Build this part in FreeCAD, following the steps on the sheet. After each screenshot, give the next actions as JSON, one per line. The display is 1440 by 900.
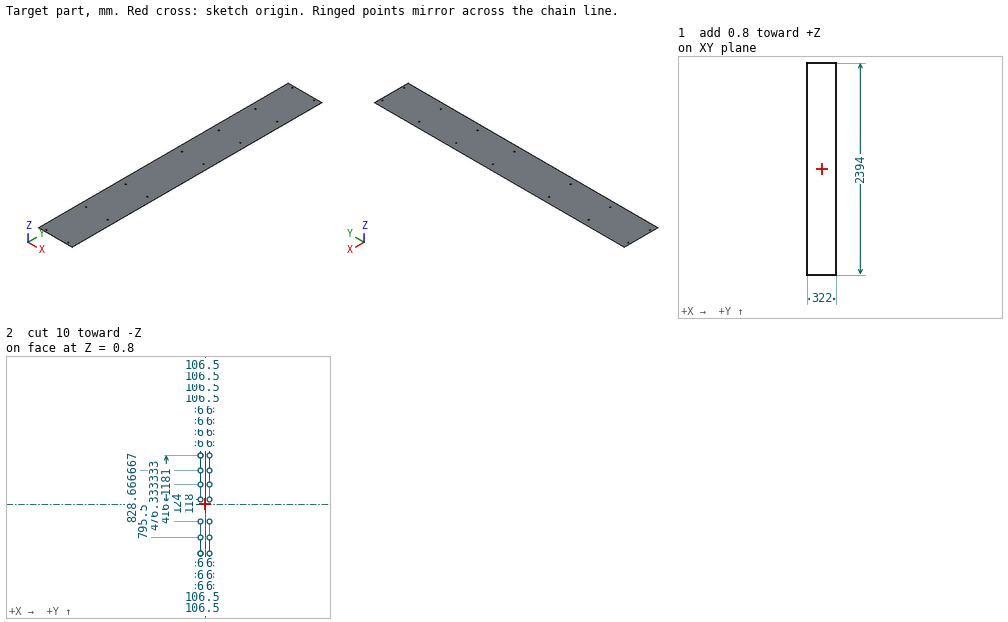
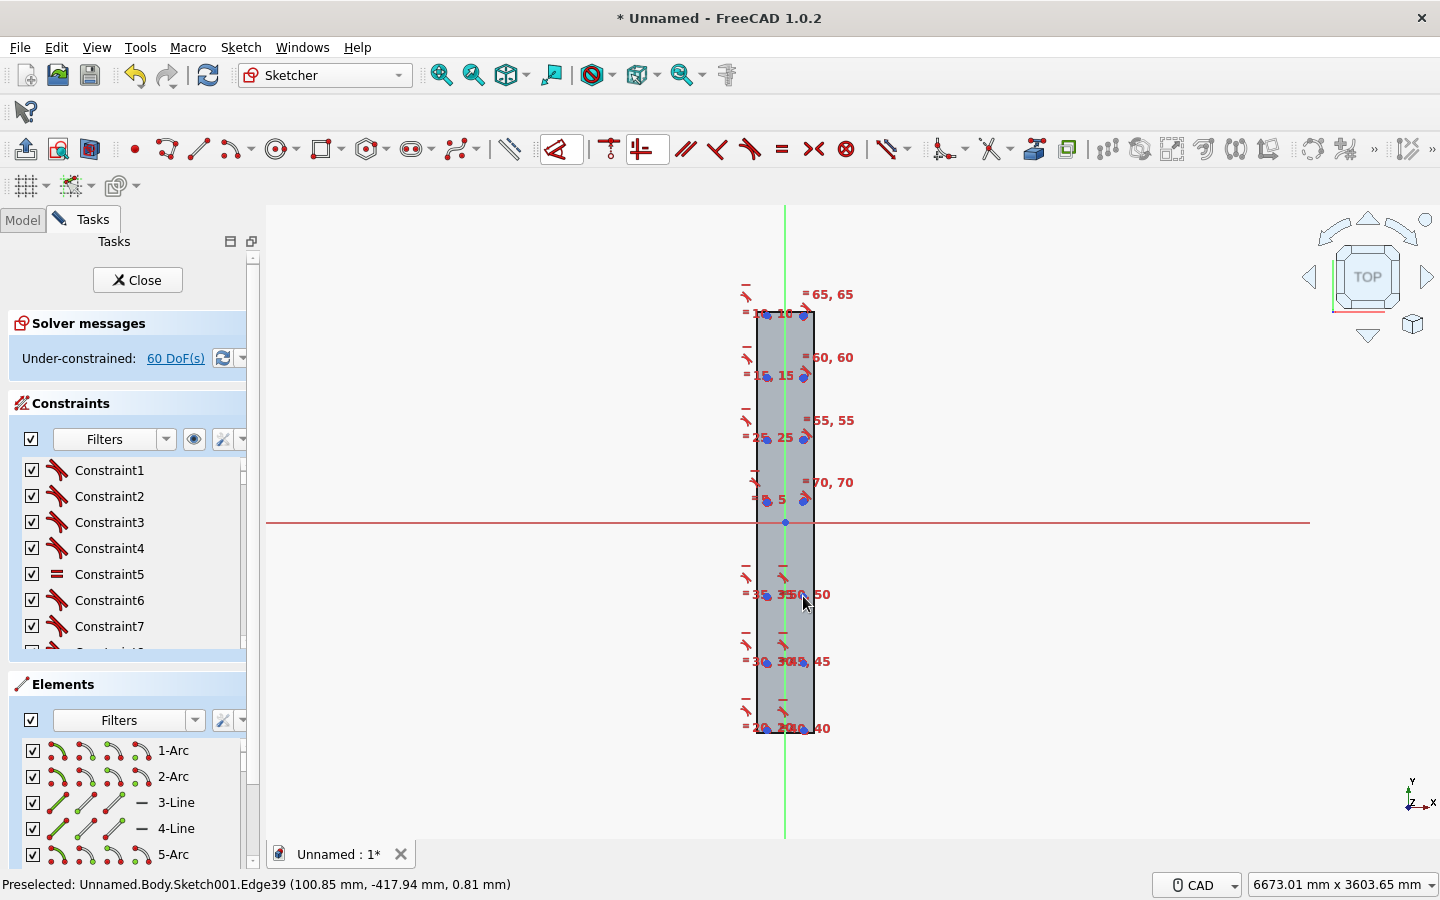
{"action": "scroll", "coordinate": [803, 439], "scroll_direction": "up", "scroll_amount": 14}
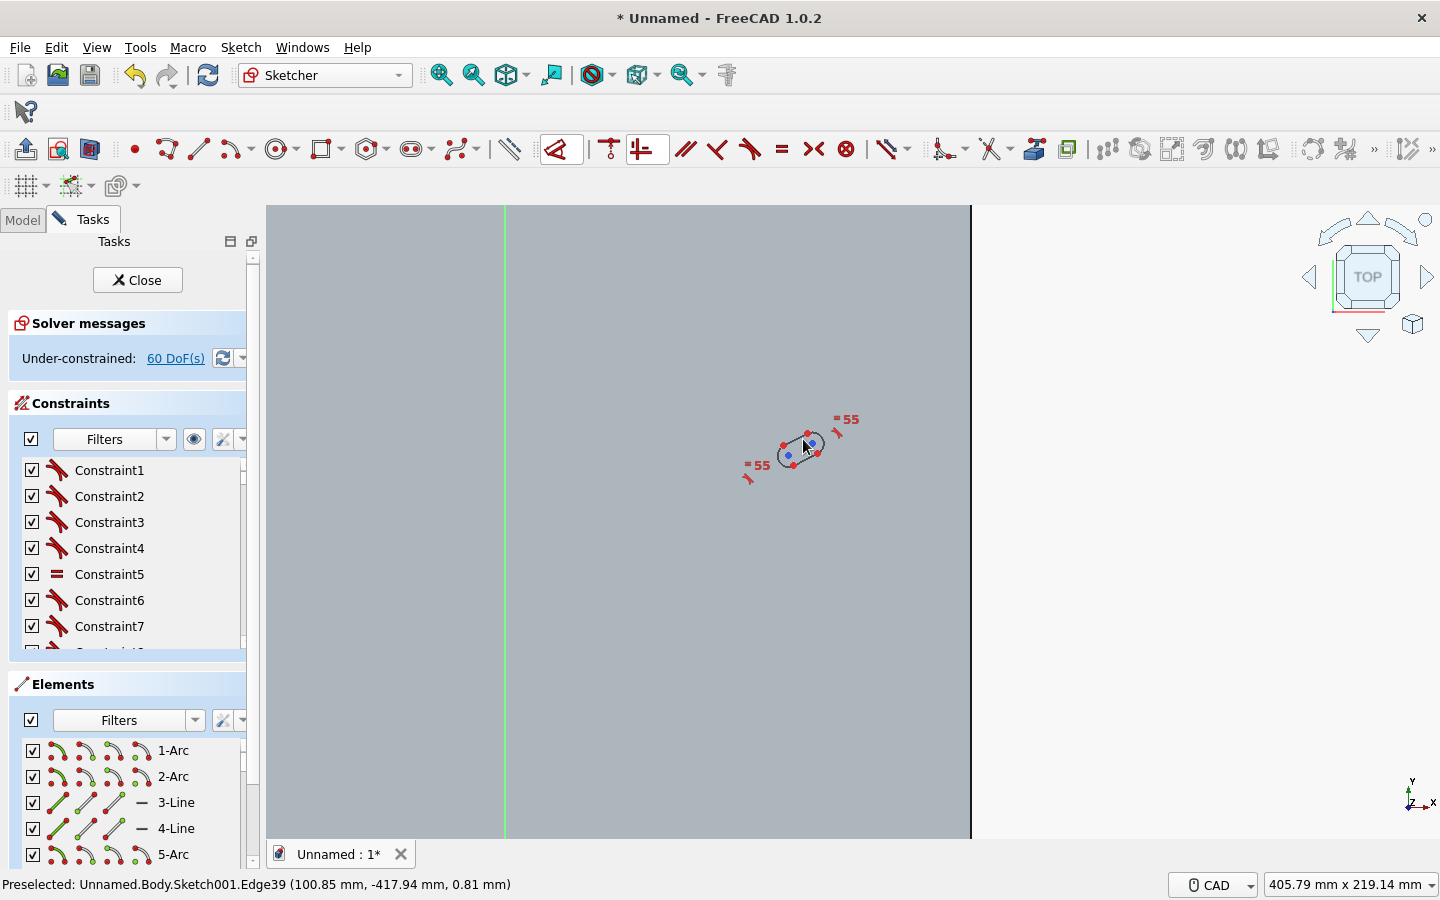
{"action": "left_click", "coordinate": [793, 441]}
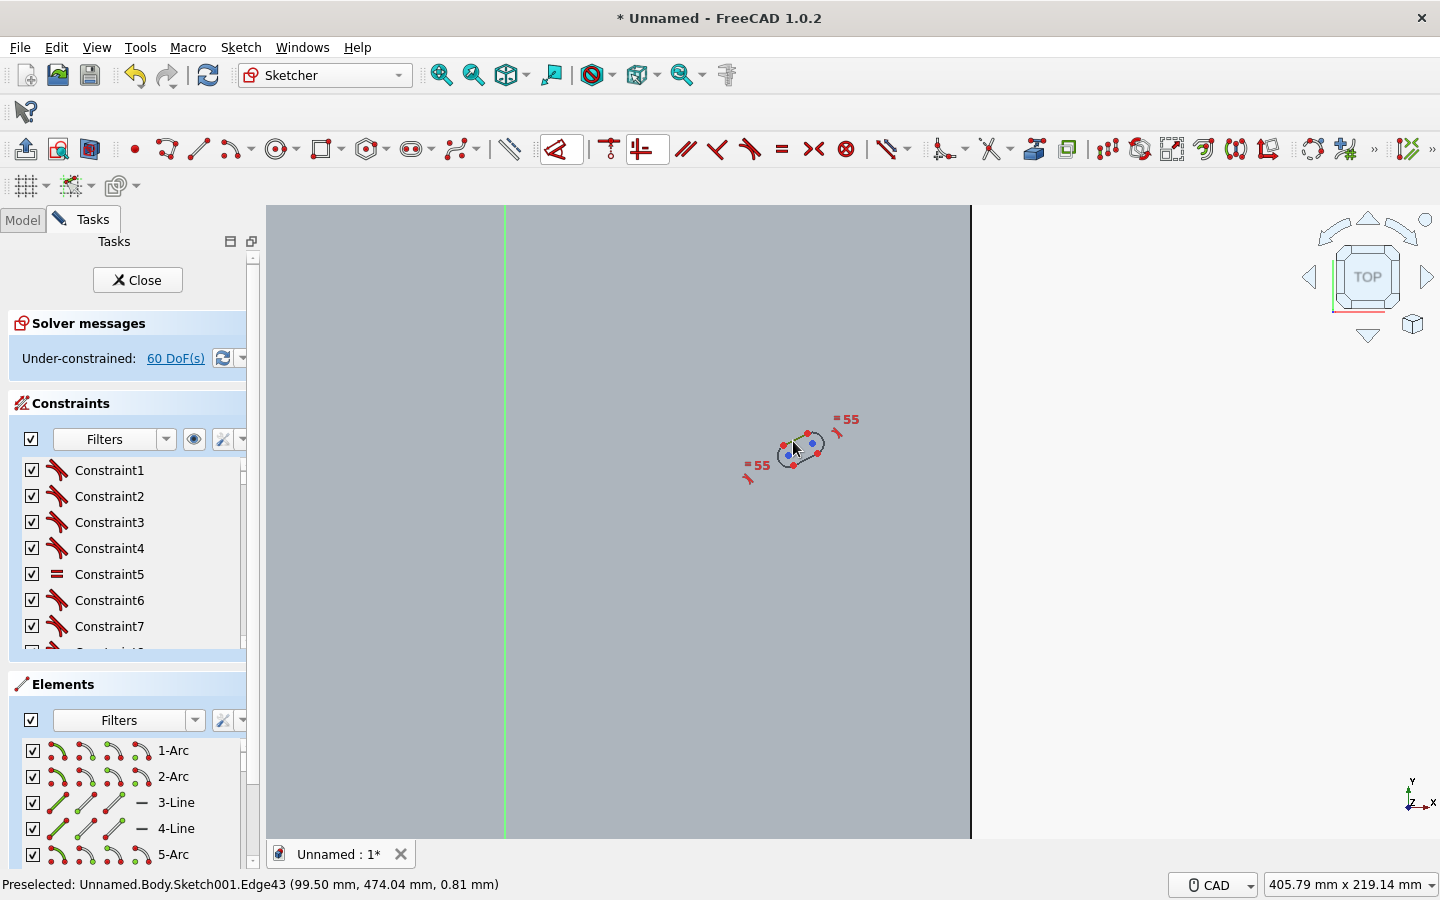
{"action": "left_click", "coordinate": [664, 150]}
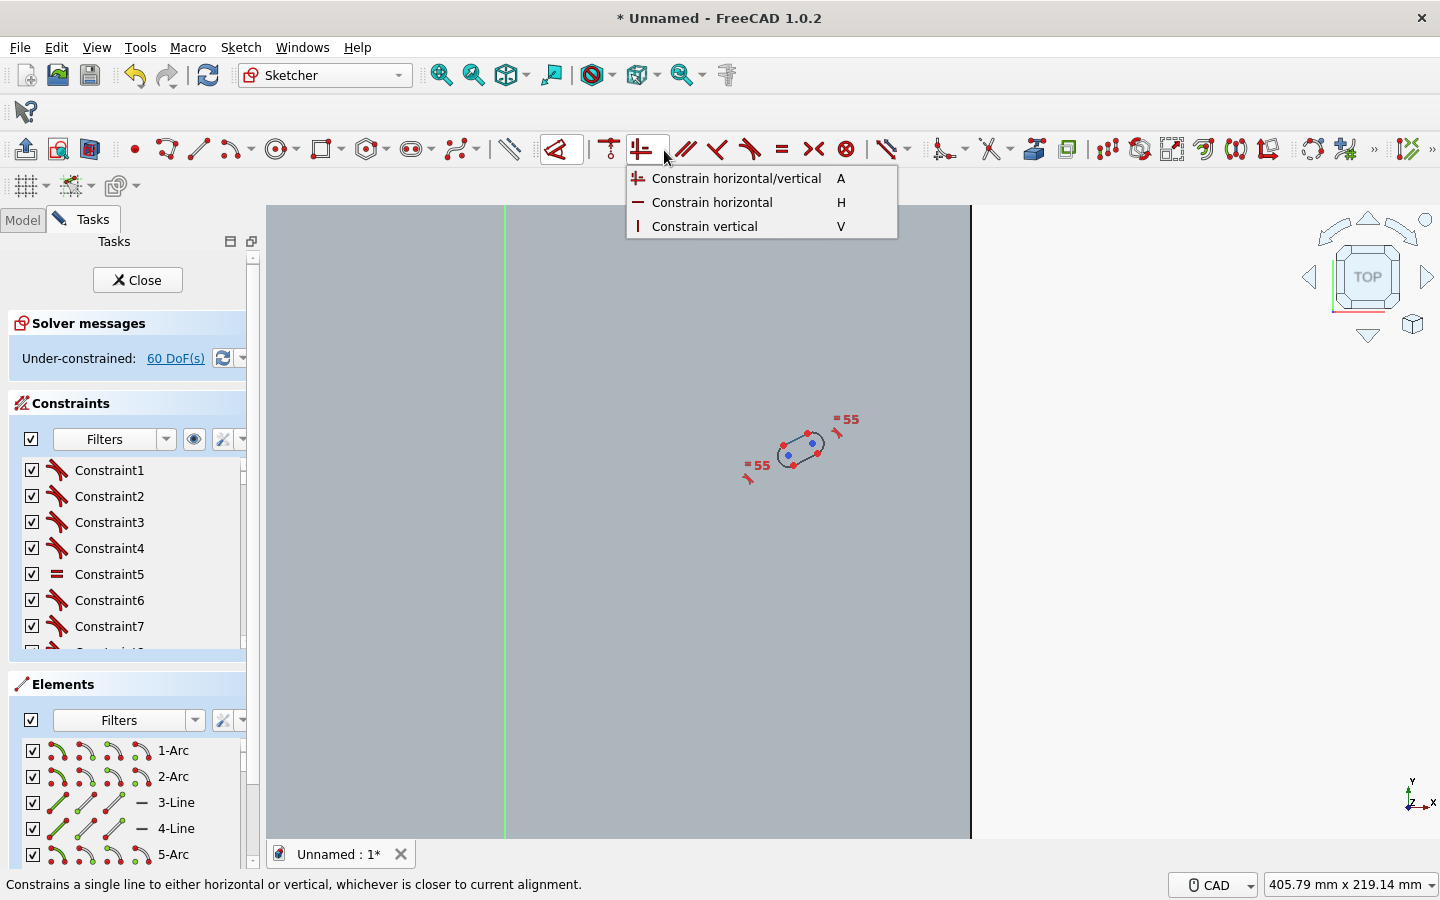
{"action": "left_click", "coordinate": [762, 202]}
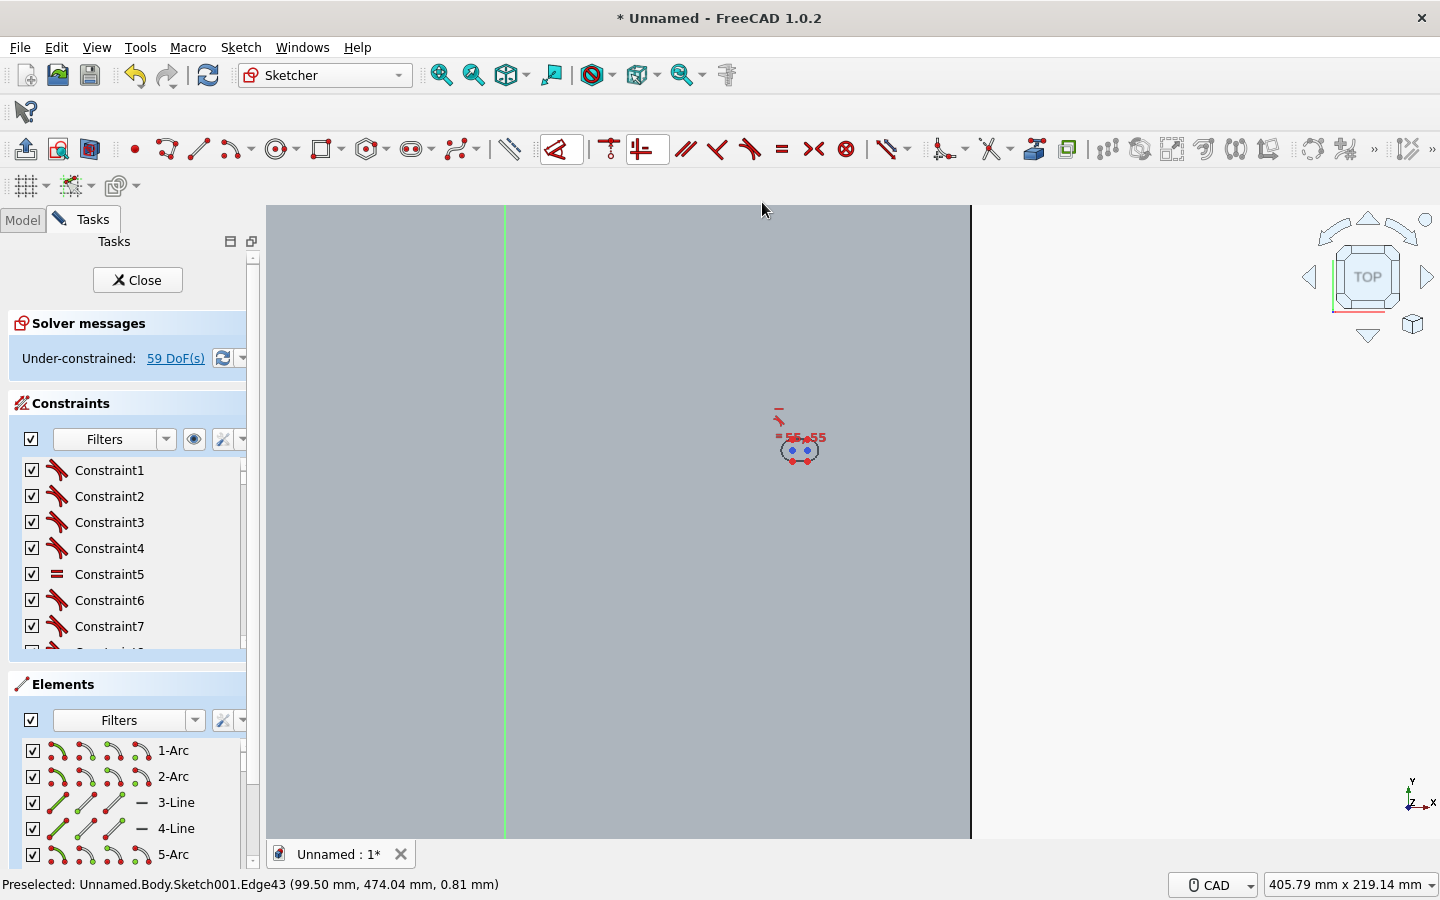
{"action": "scroll", "coordinate": [803, 438], "scroll_direction": "down", "scroll_amount": 14}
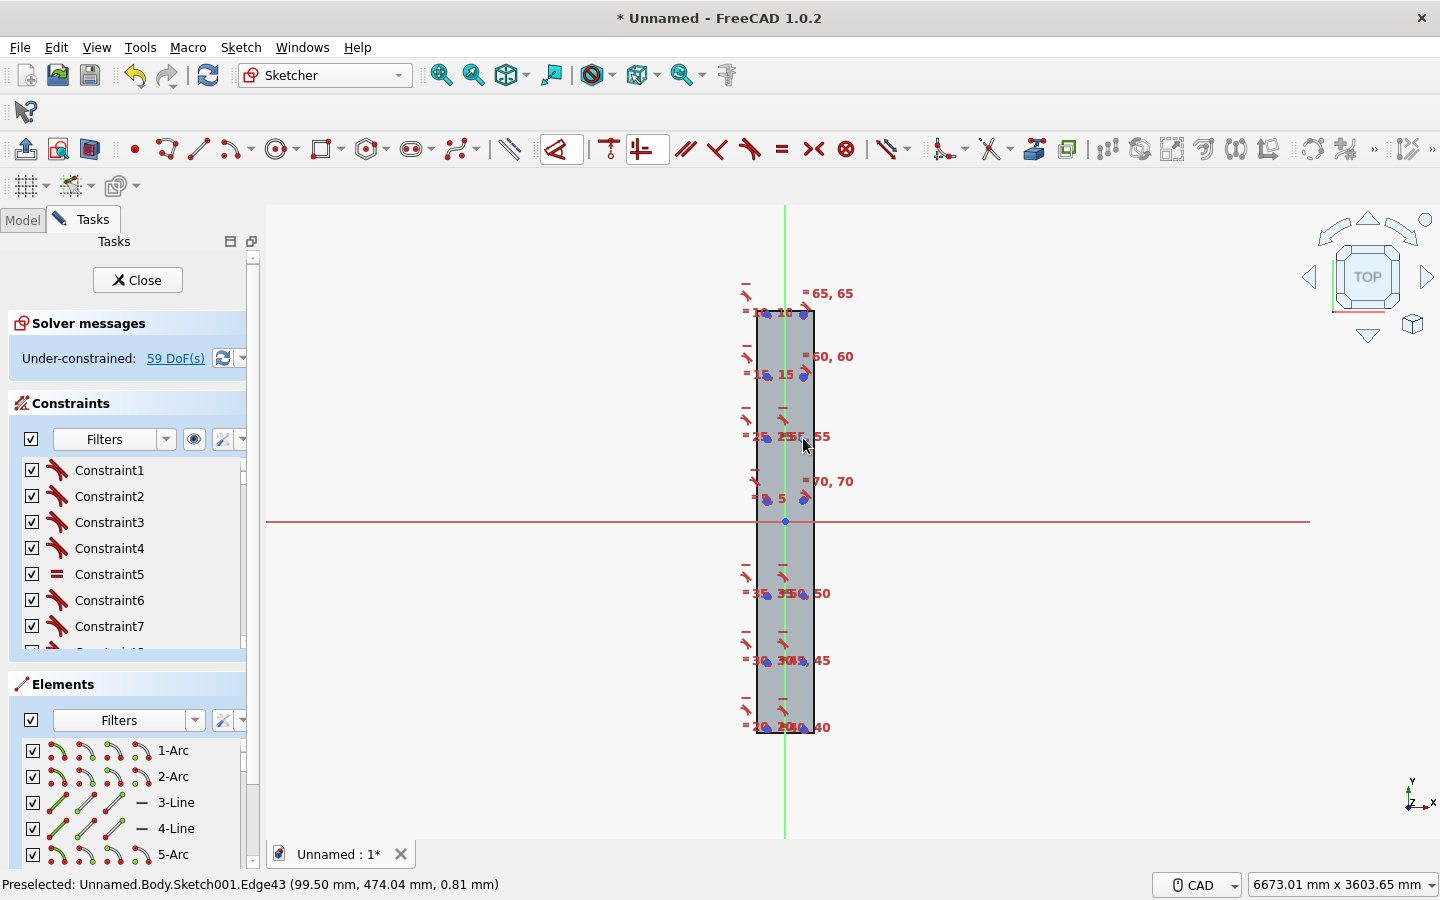
{"action": "scroll", "coordinate": [803, 377], "scroll_direction": "up", "scroll_amount": 14}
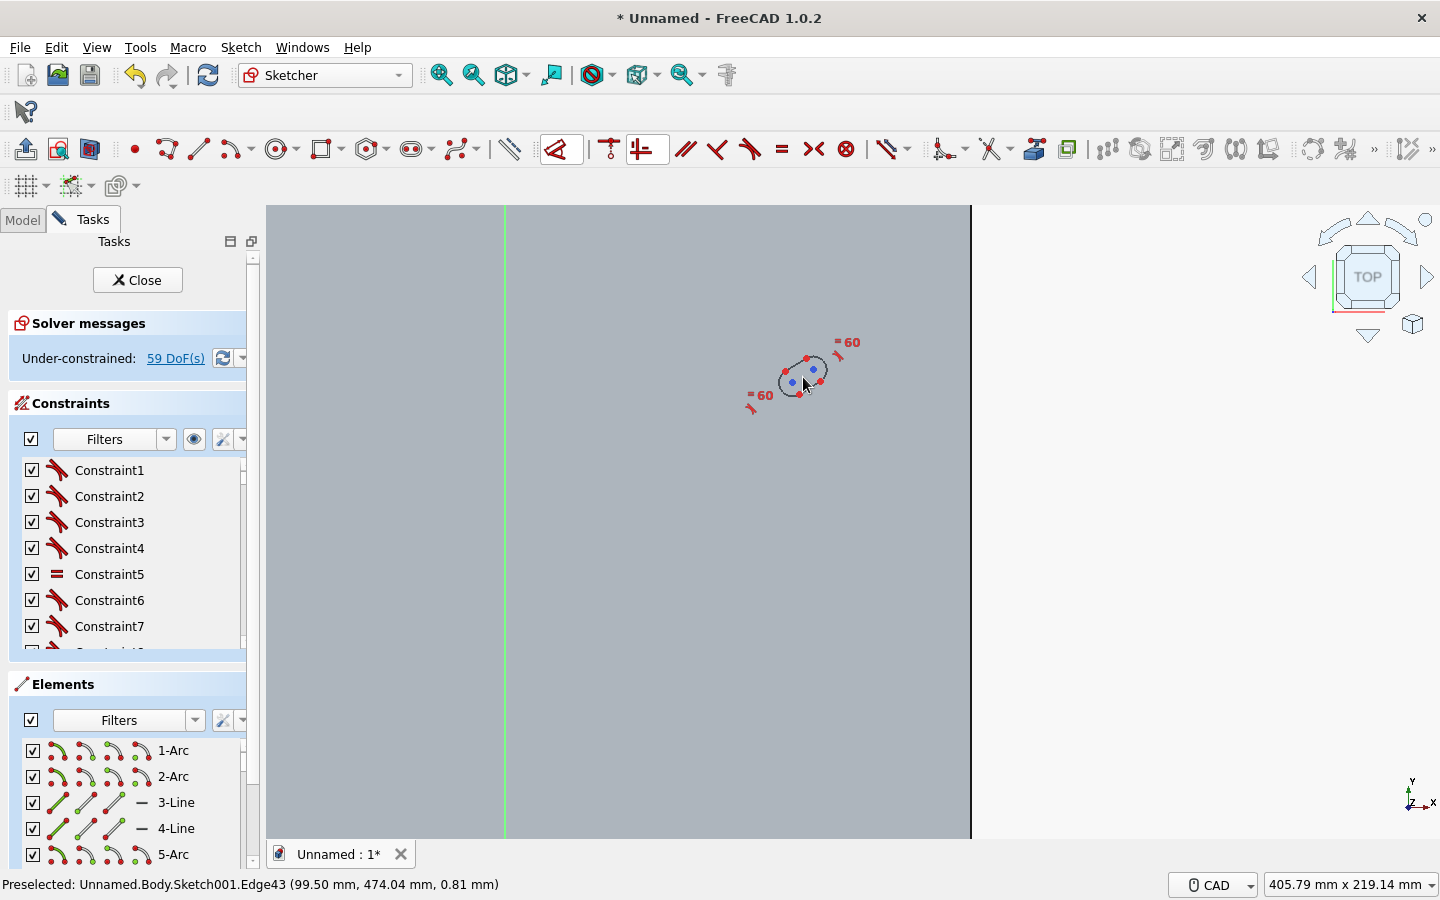
{"action": "left_click", "coordinate": [794, 366]}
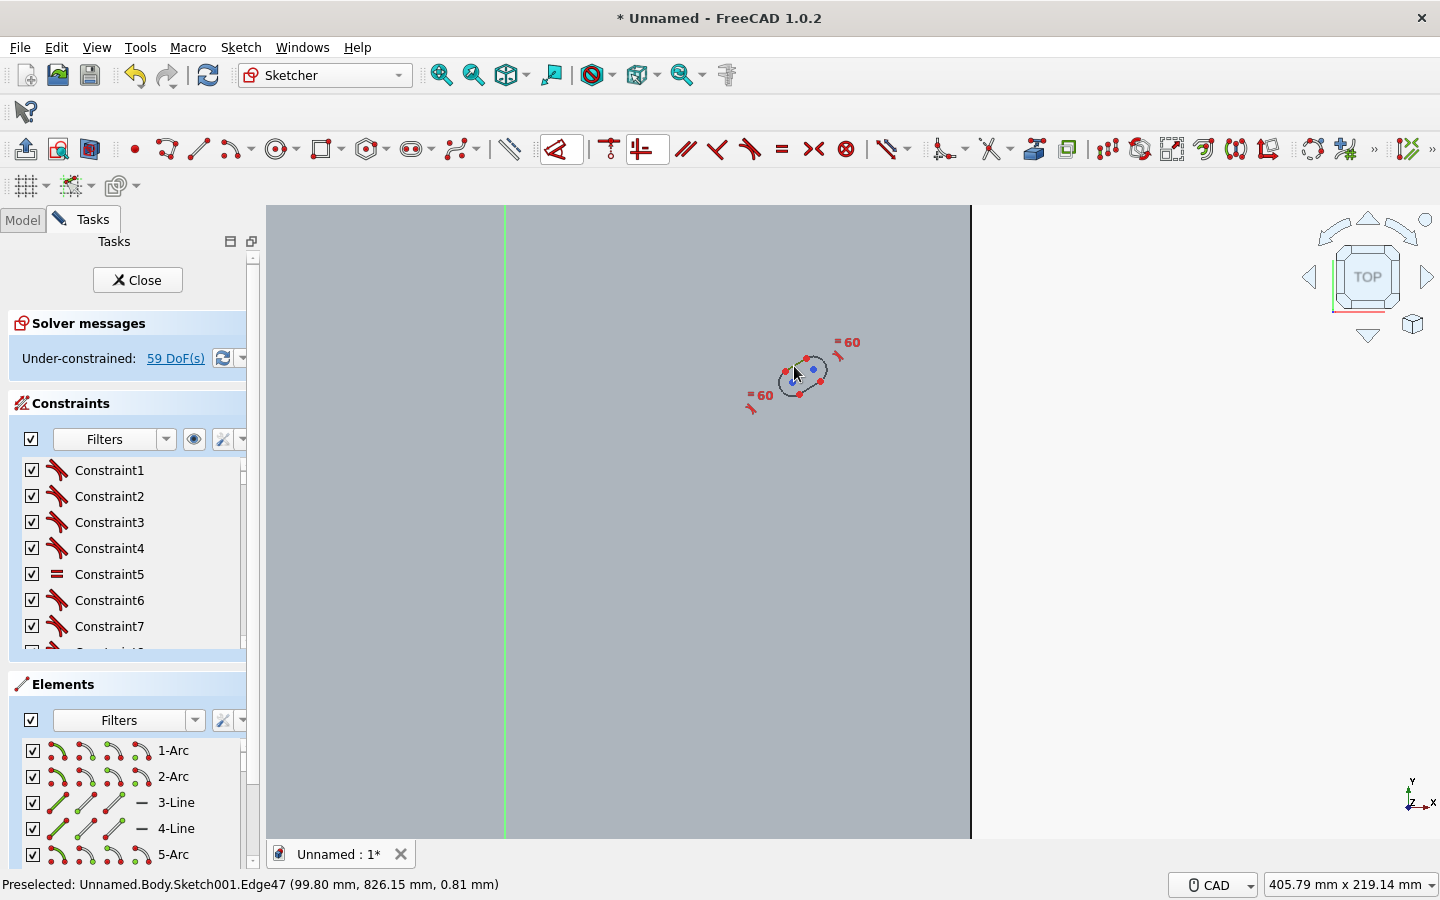
{"action": "key", "text": "h"}